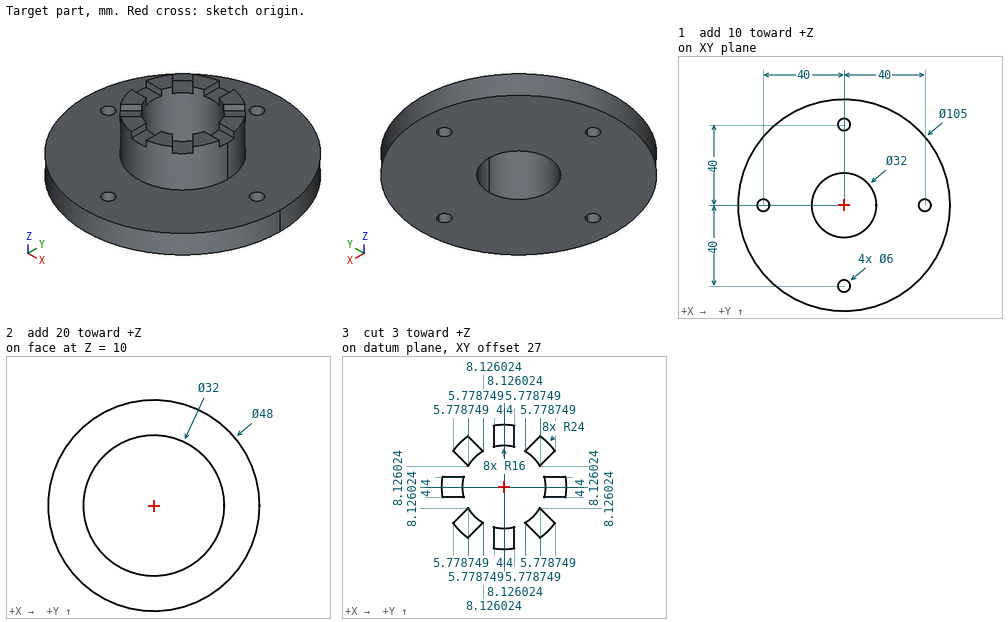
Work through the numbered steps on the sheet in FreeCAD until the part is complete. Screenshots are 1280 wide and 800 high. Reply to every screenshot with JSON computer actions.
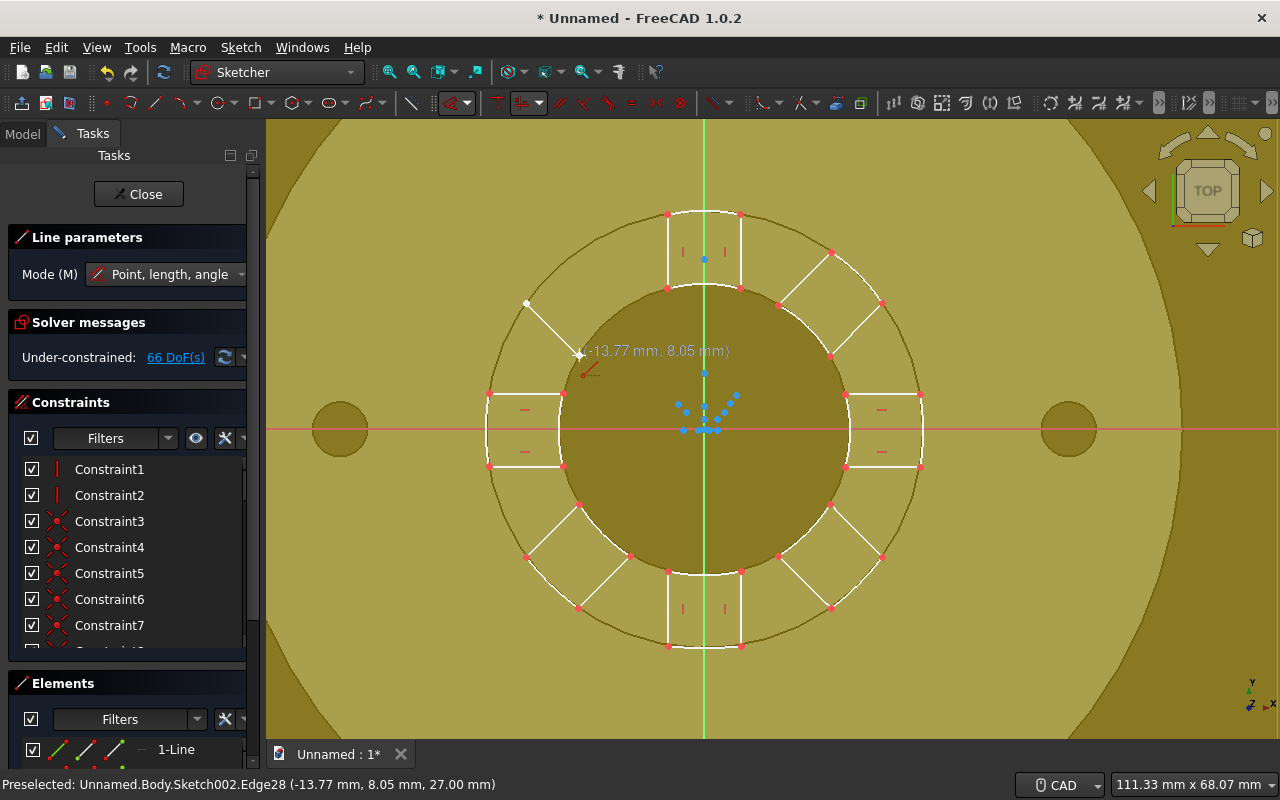
{"action": "left_click", "coordinate": [630, 304]}
{"action": "left_click", "coordinate": [578, 251]}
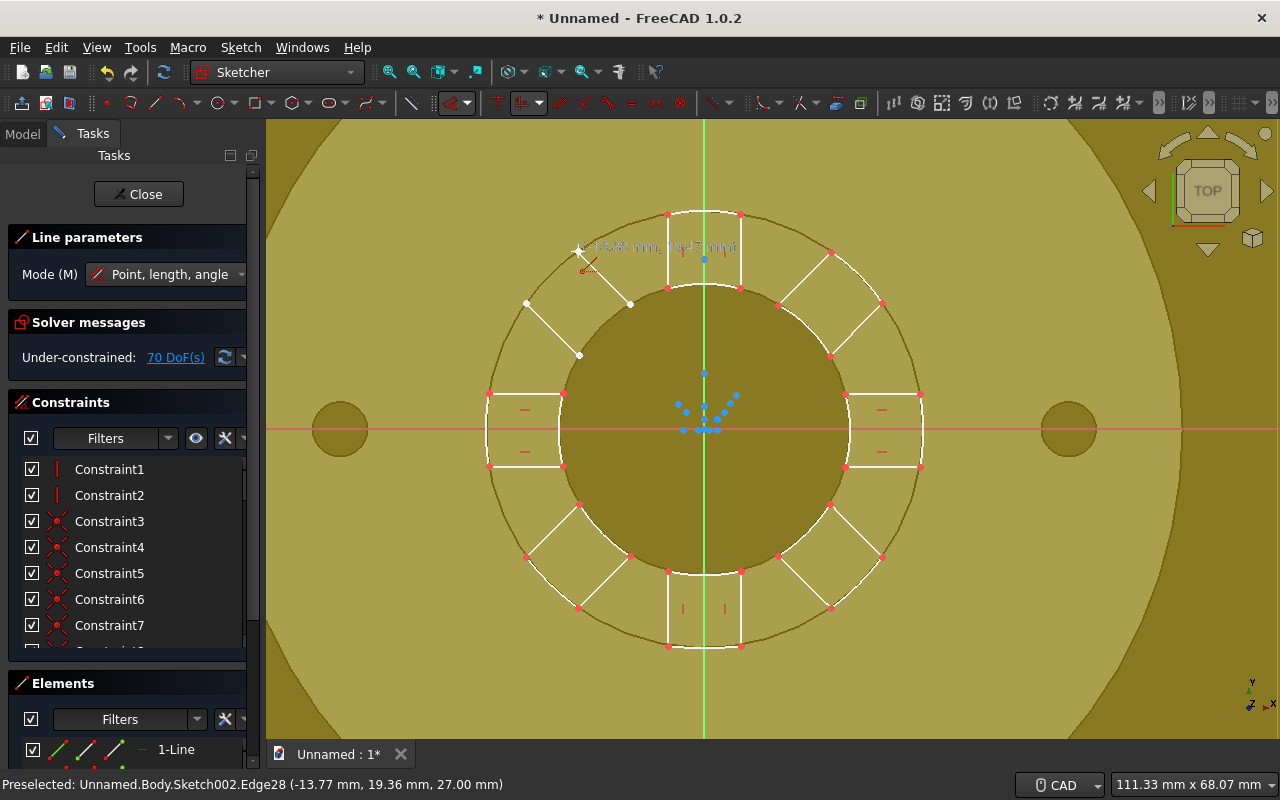
{"action": "left_click", "coordinate": [180, 104]}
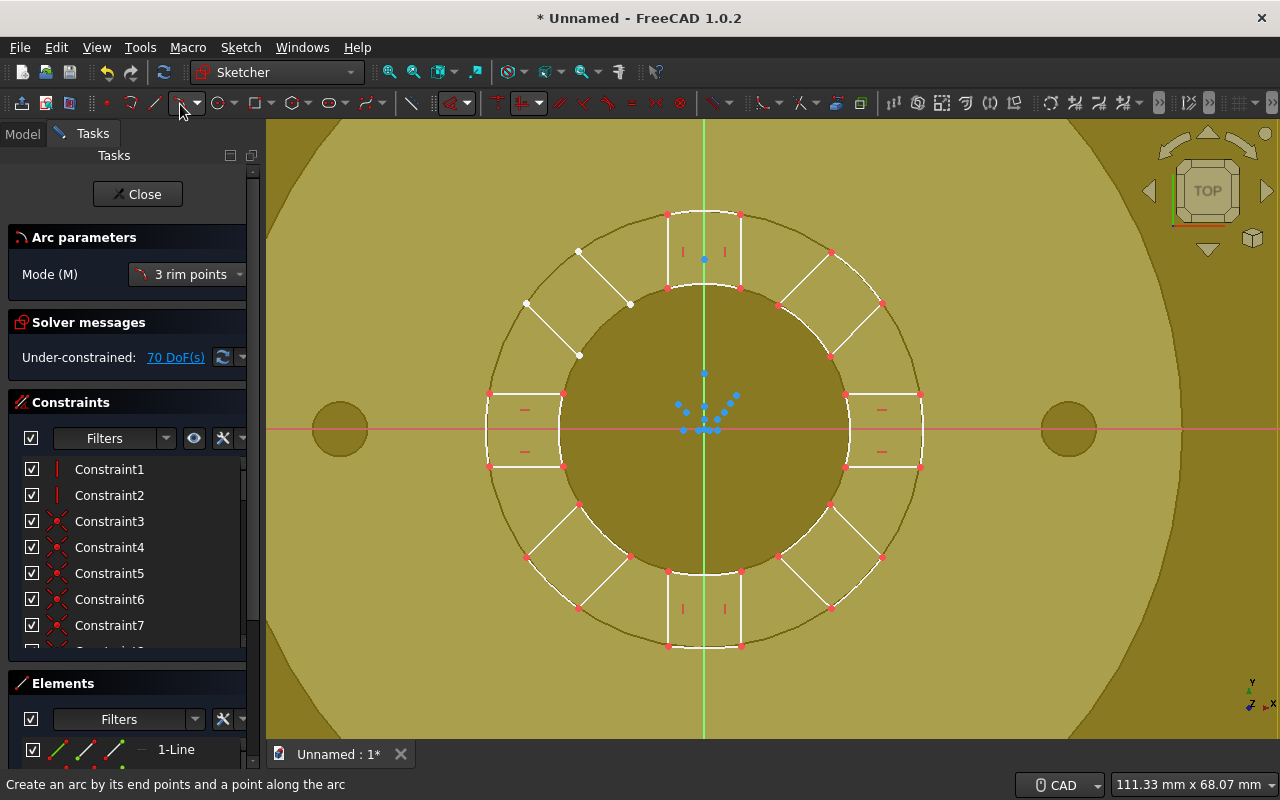
{"action": "left_click", "coordinate": [579, 356]}
{"action": "left_click", "coordinate": [630, 305]}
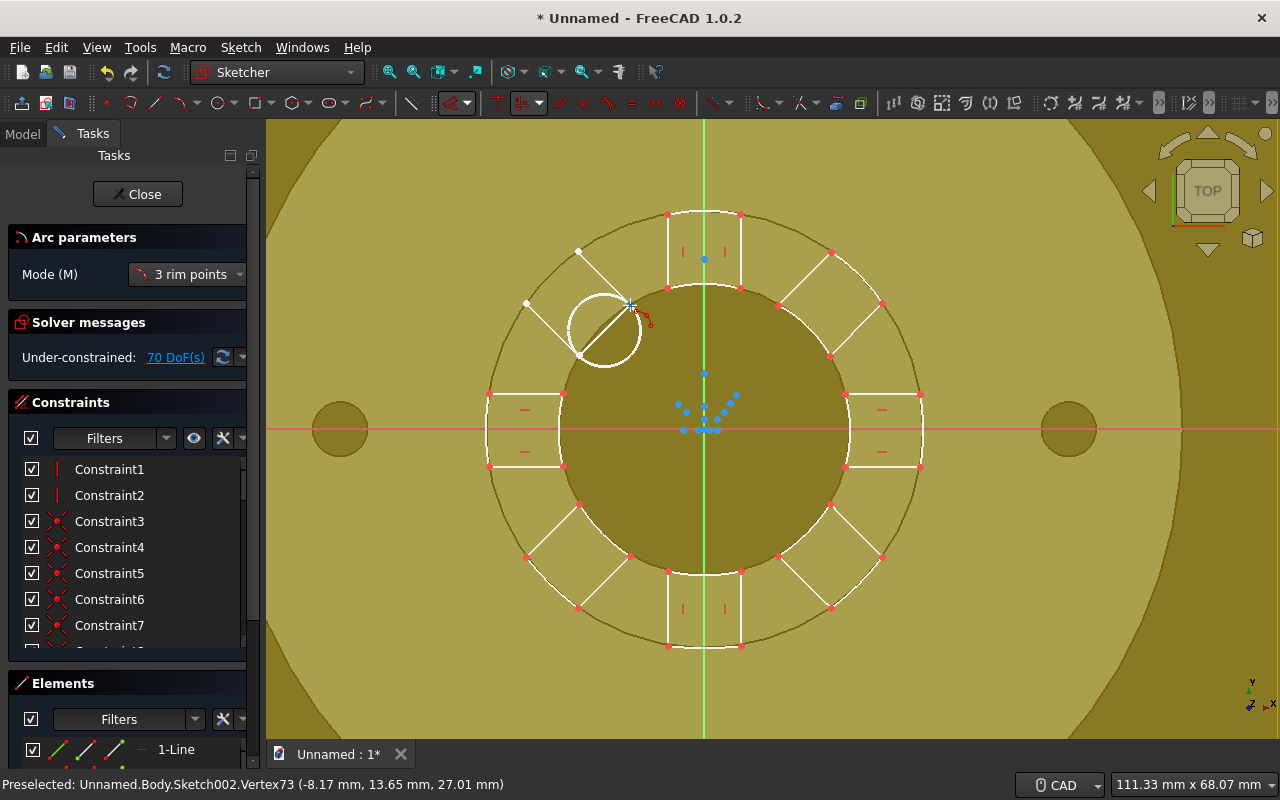
{"action": "scroll", "coordinate": [601, 326], "scroll_direction": "up", "scroll_amount": 7}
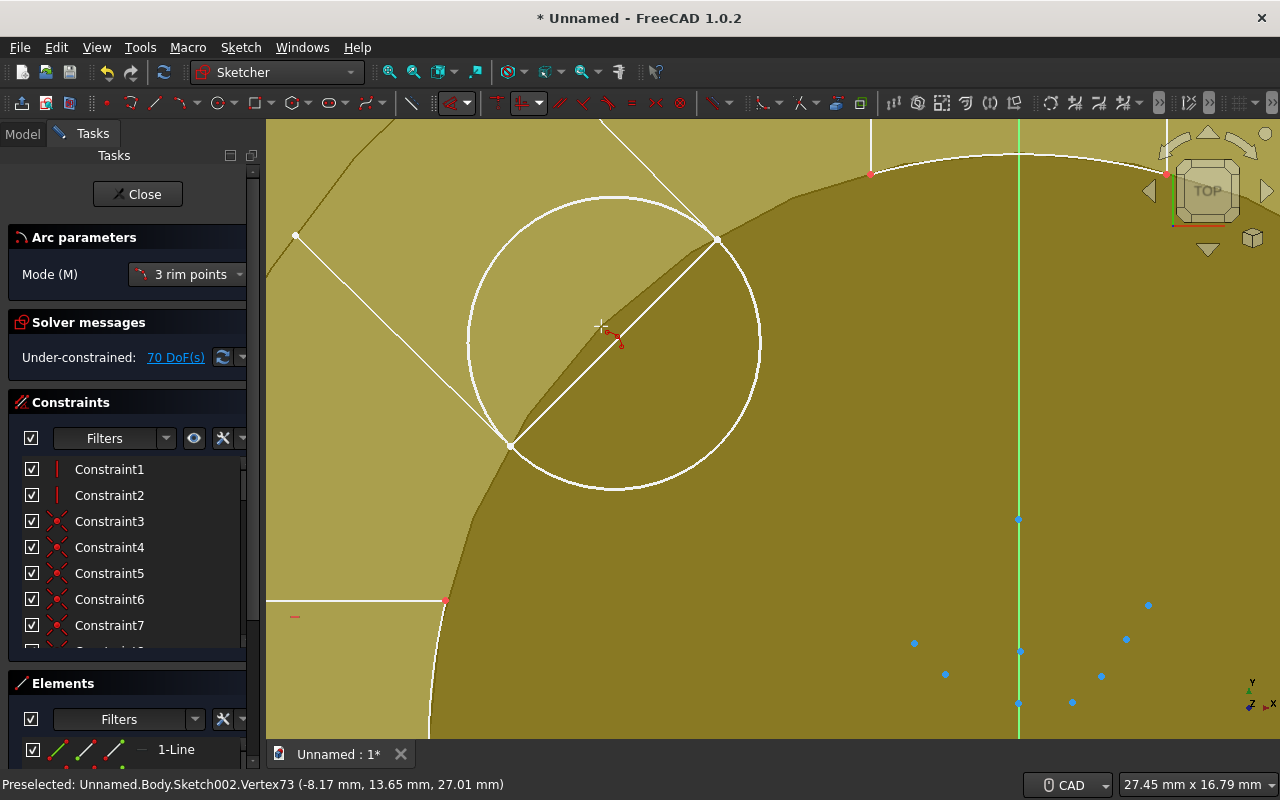
{"action": "left_click", "coordinate": [602, 326]}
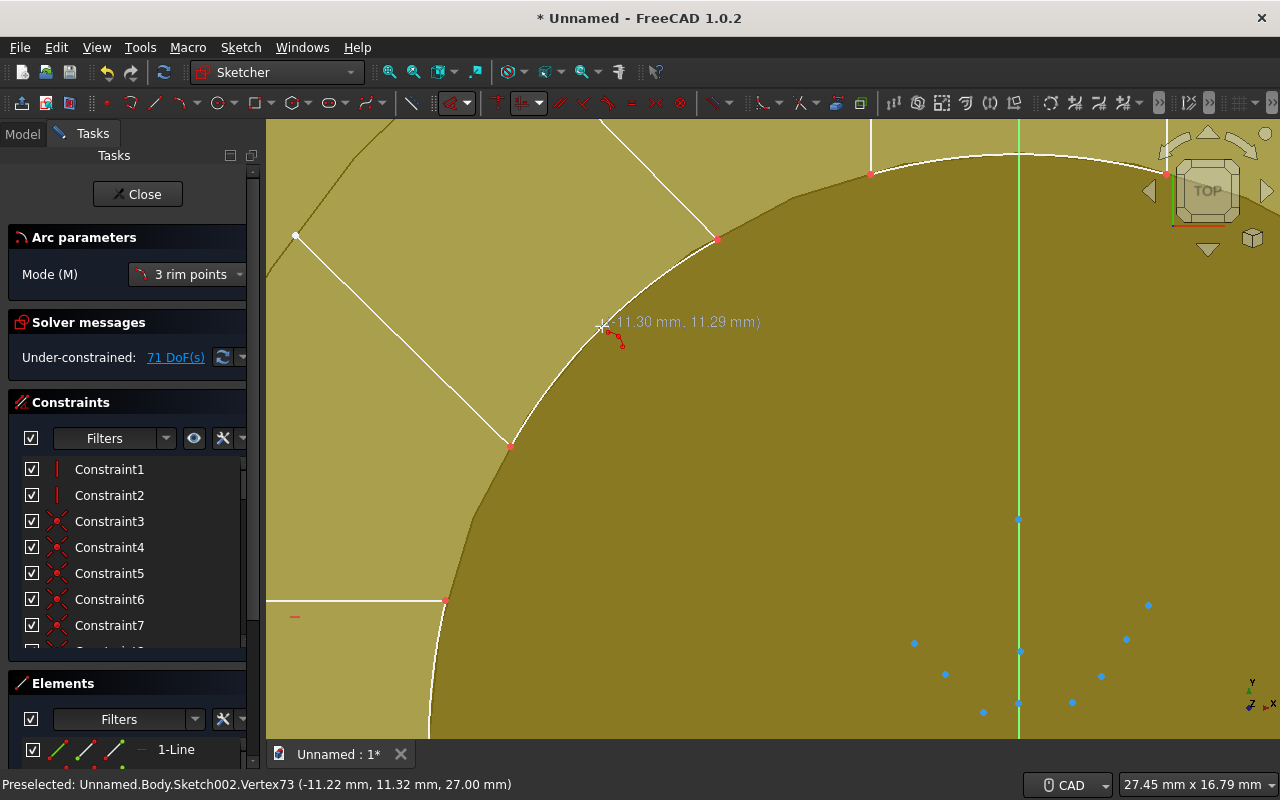
{"action": "scroll", "coordinate": [601, 326], "scroll_direction": "down", "scroll_amount": 7}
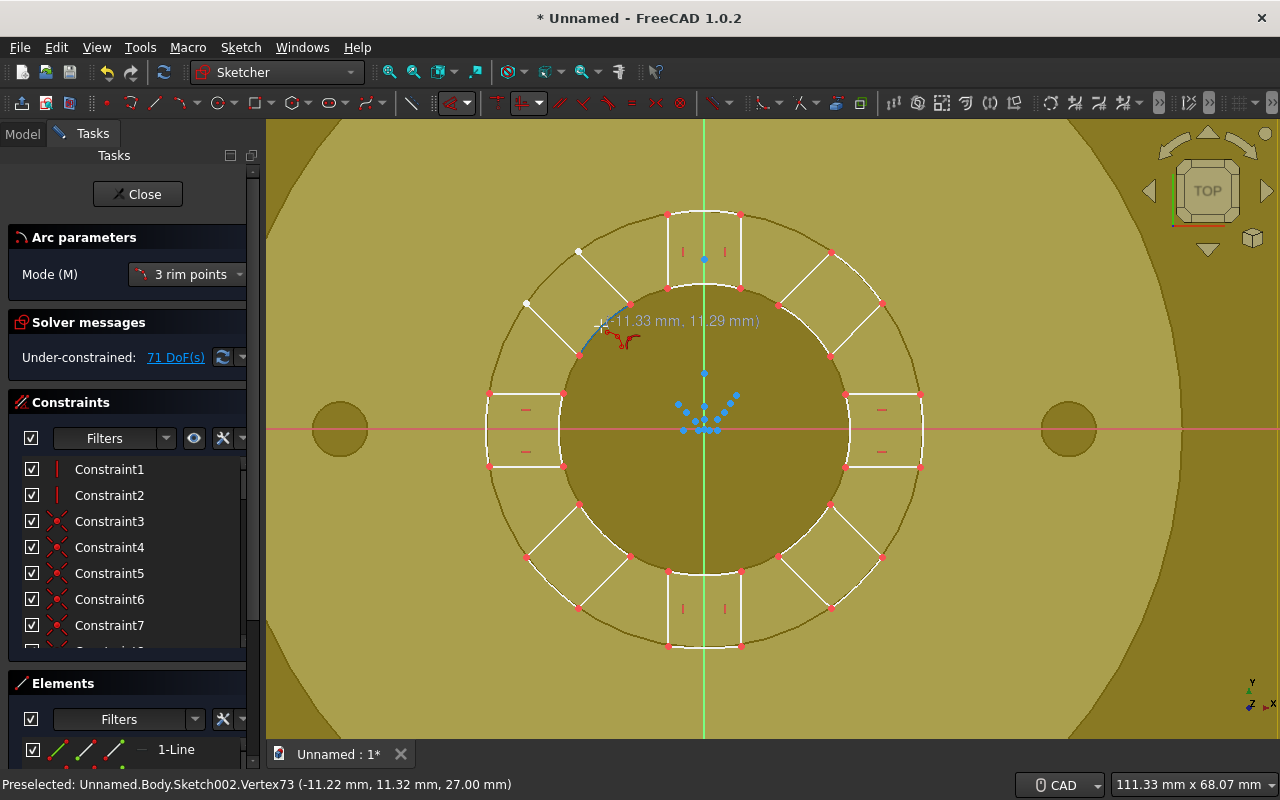
{"action": "left_click", "coordinate": [578, 252]}
{"action": "left_click", "coordinate": [526, 304]}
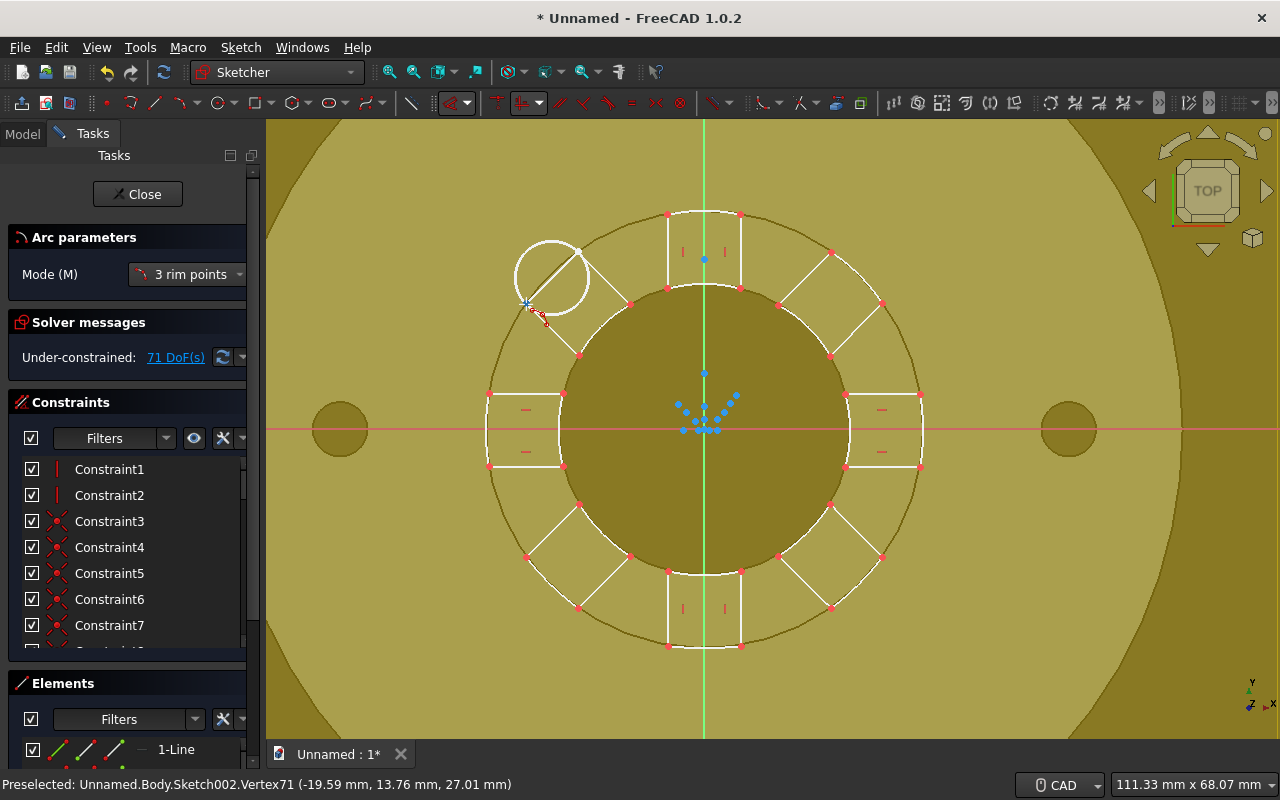
{"action": "scroll", "coordinate": [550, 275], "scroll_direction": "up", "scroll_amount": 9}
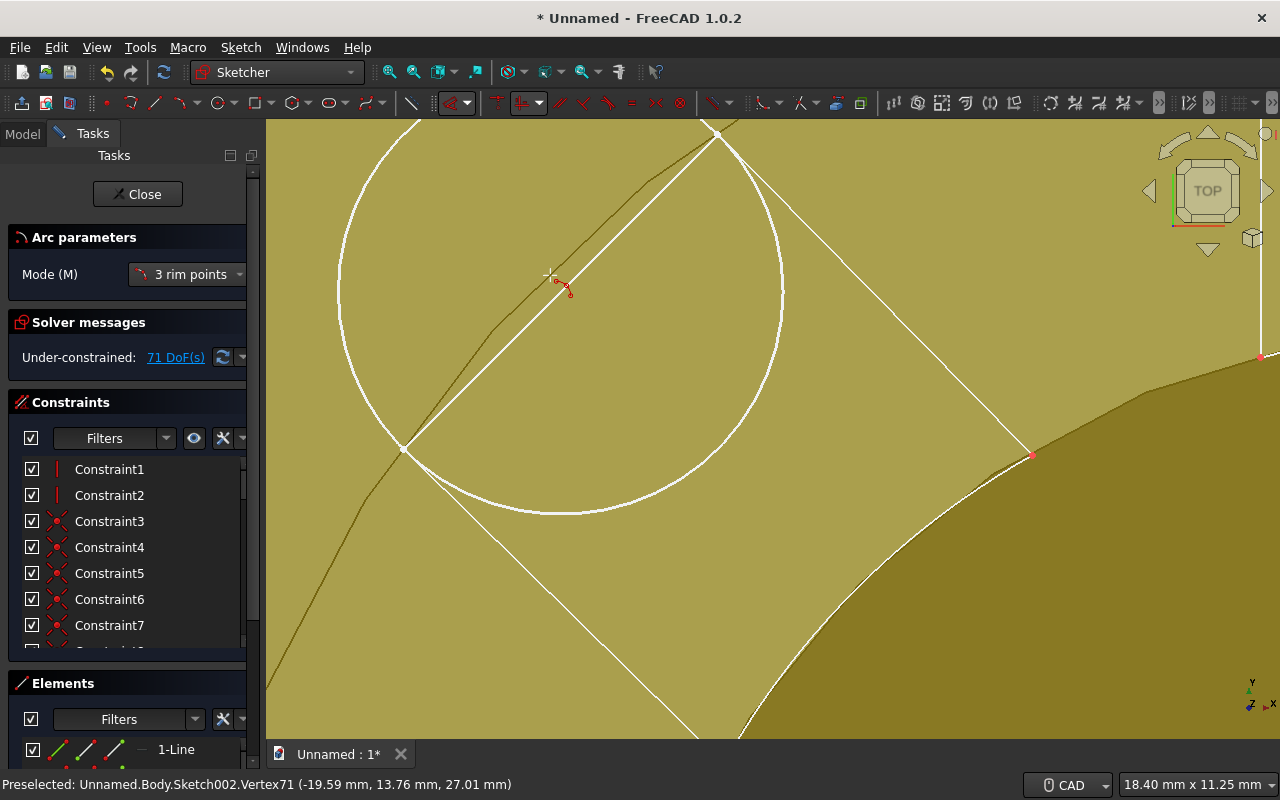
{"action": "left_click", "coordinate": [548, 272]}
{"action": "key", "text": "Escape"}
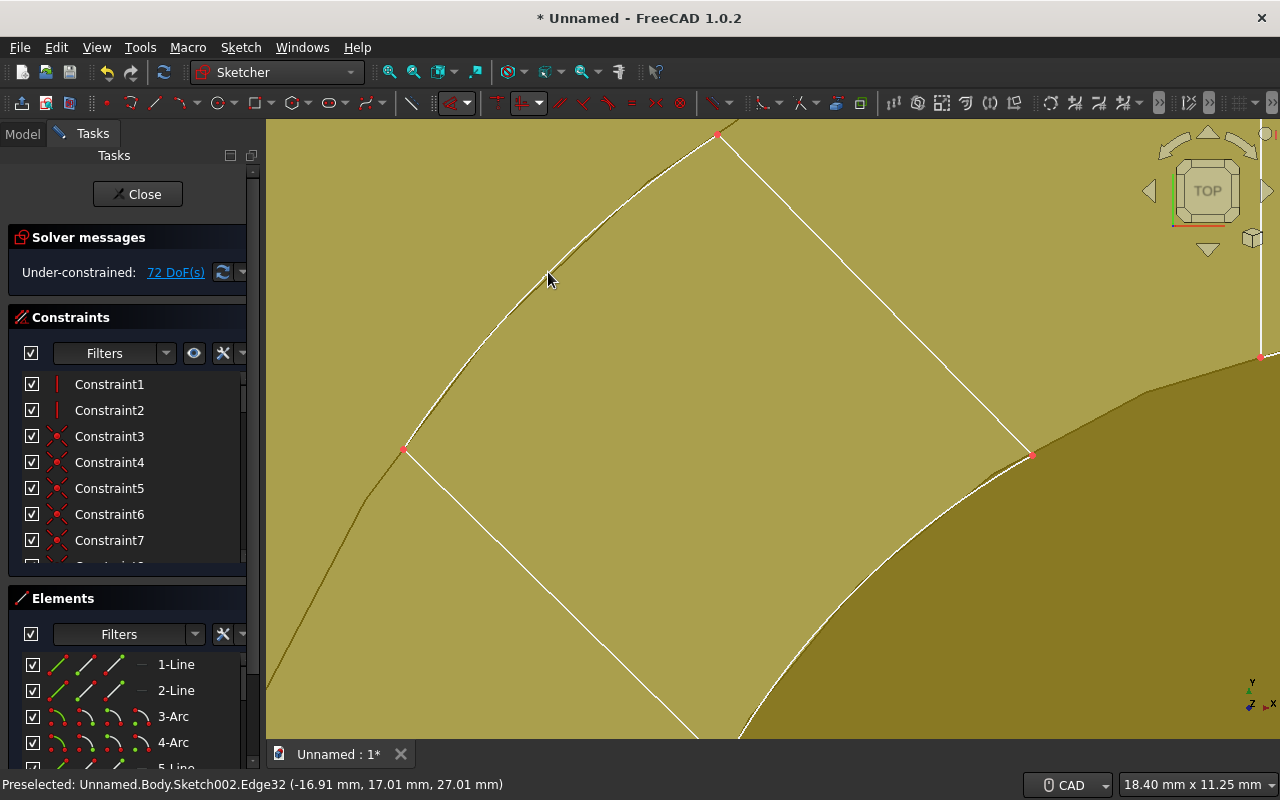
{"action": "scroll", "coordinate": [550, 275], "scroll_direction": "down", "scroll_amount": 9}